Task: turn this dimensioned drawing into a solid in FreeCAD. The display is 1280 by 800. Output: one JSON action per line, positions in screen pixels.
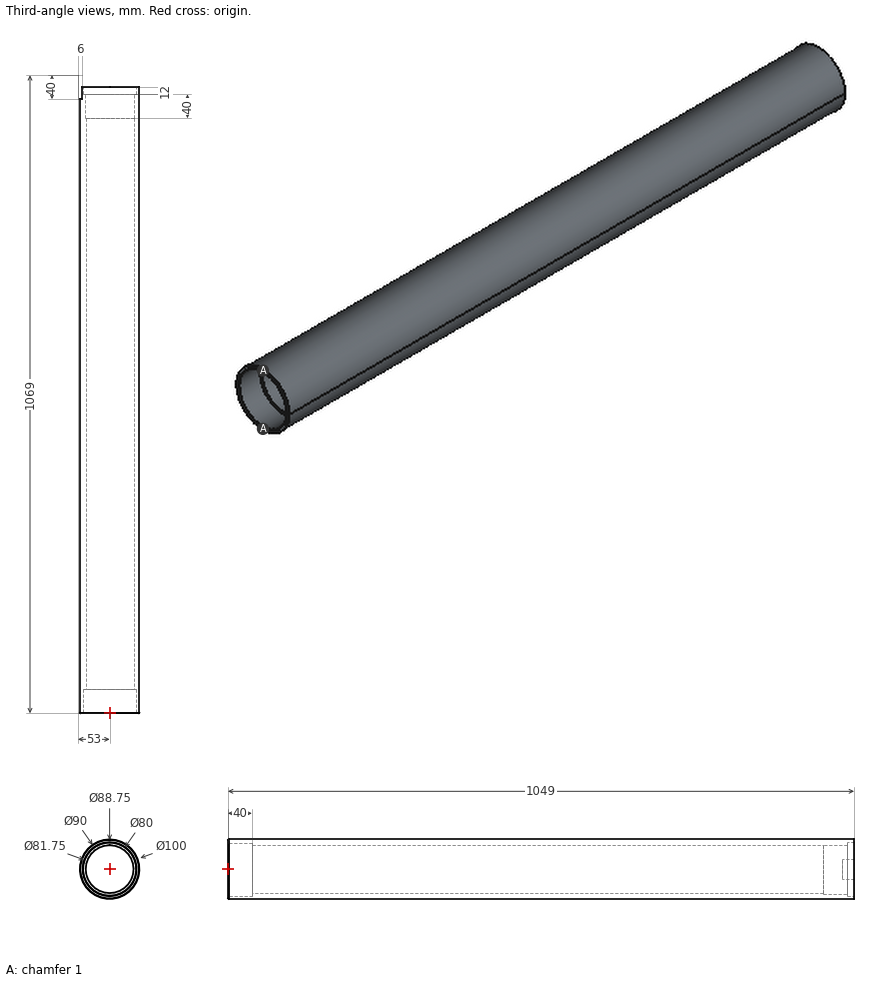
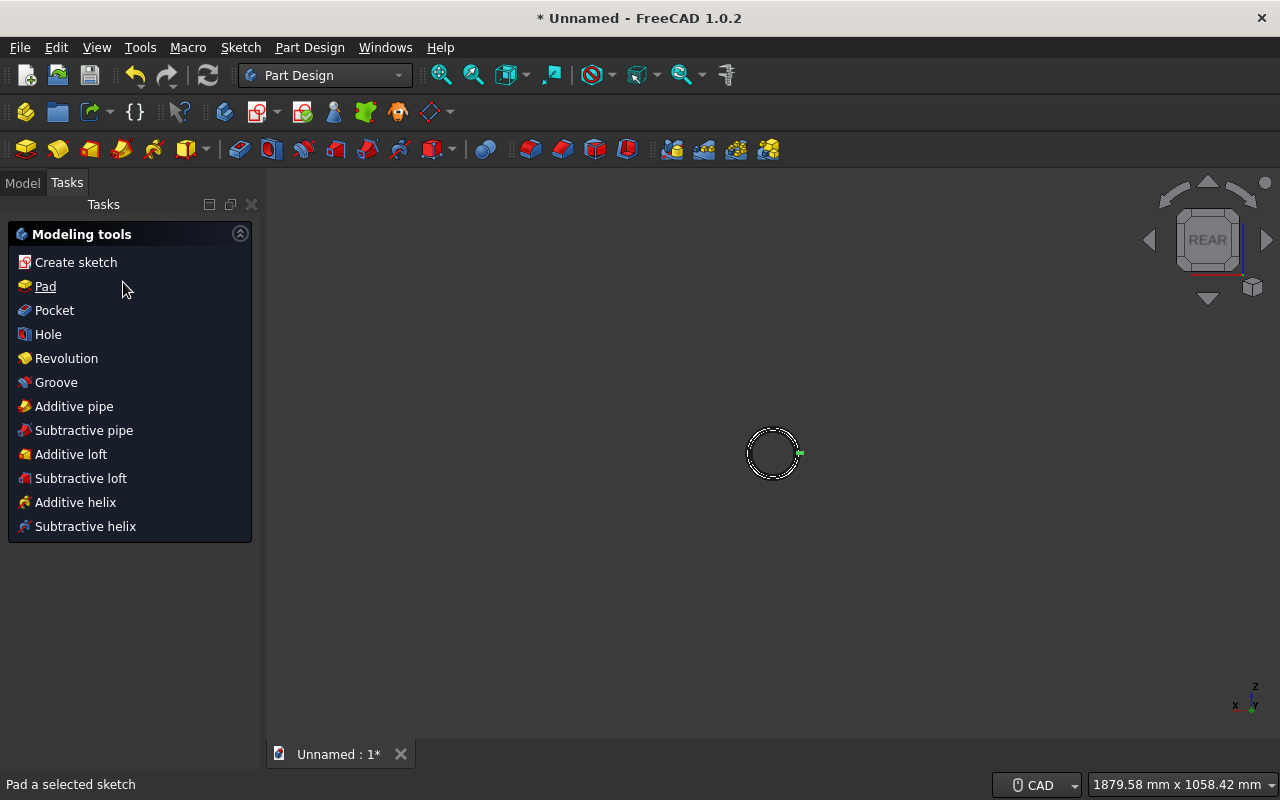
{"action": "left_click", "coordinate": [240, 150]}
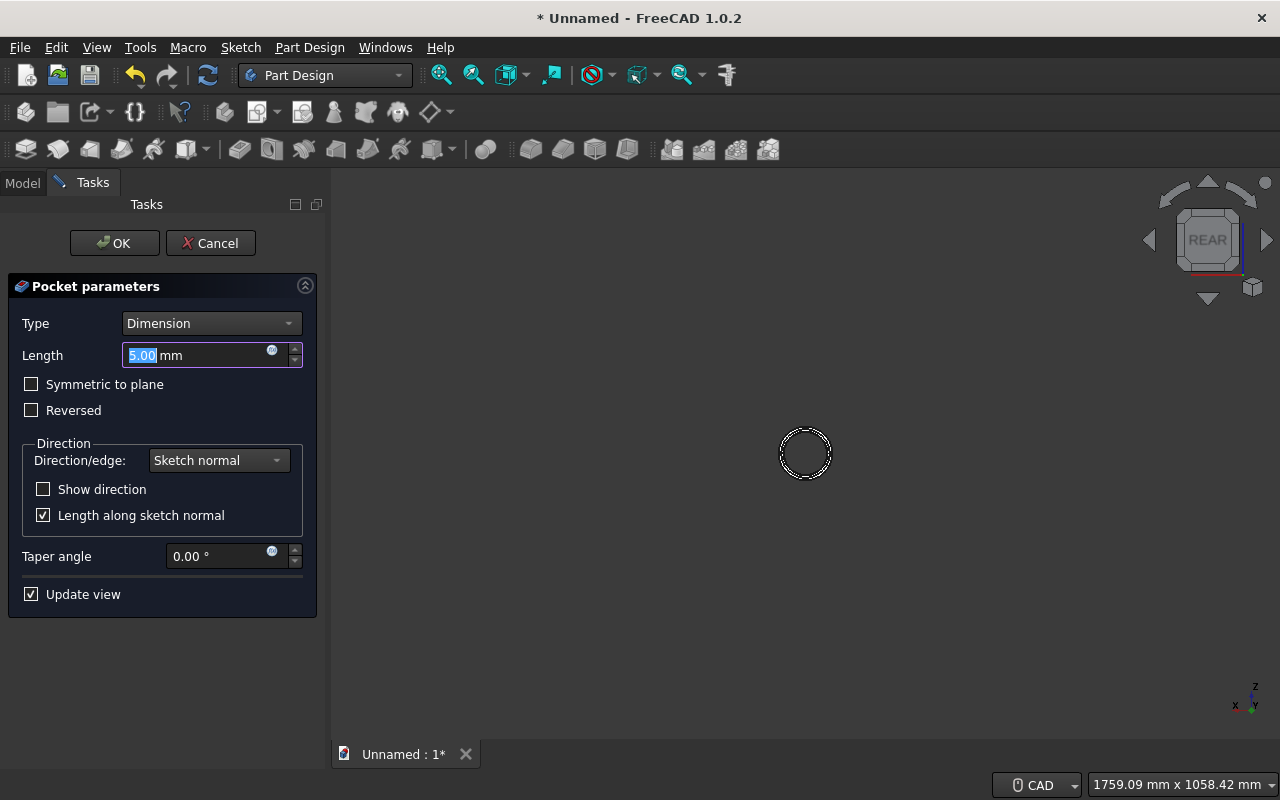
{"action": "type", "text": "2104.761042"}
{"action": "key", "text": "Tab"}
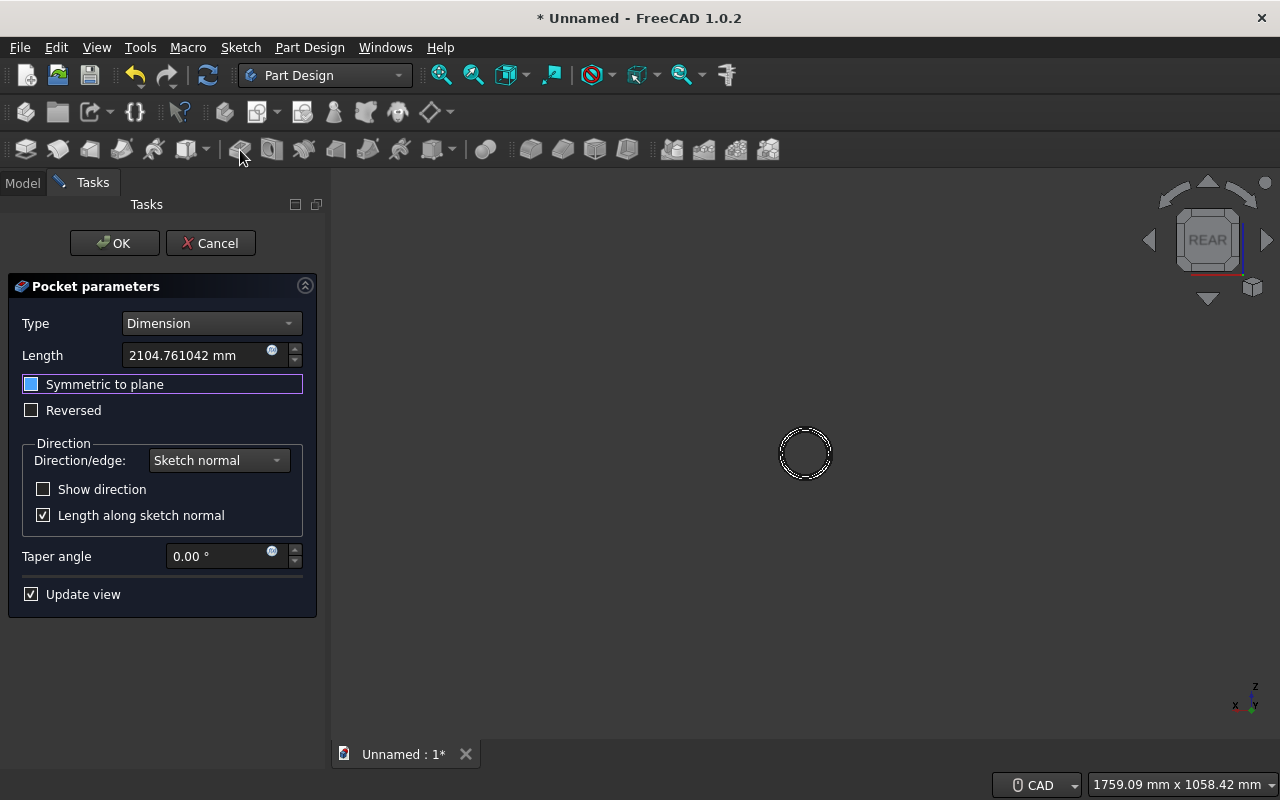
{"action": "left_click", "coordinate": [30, 384]}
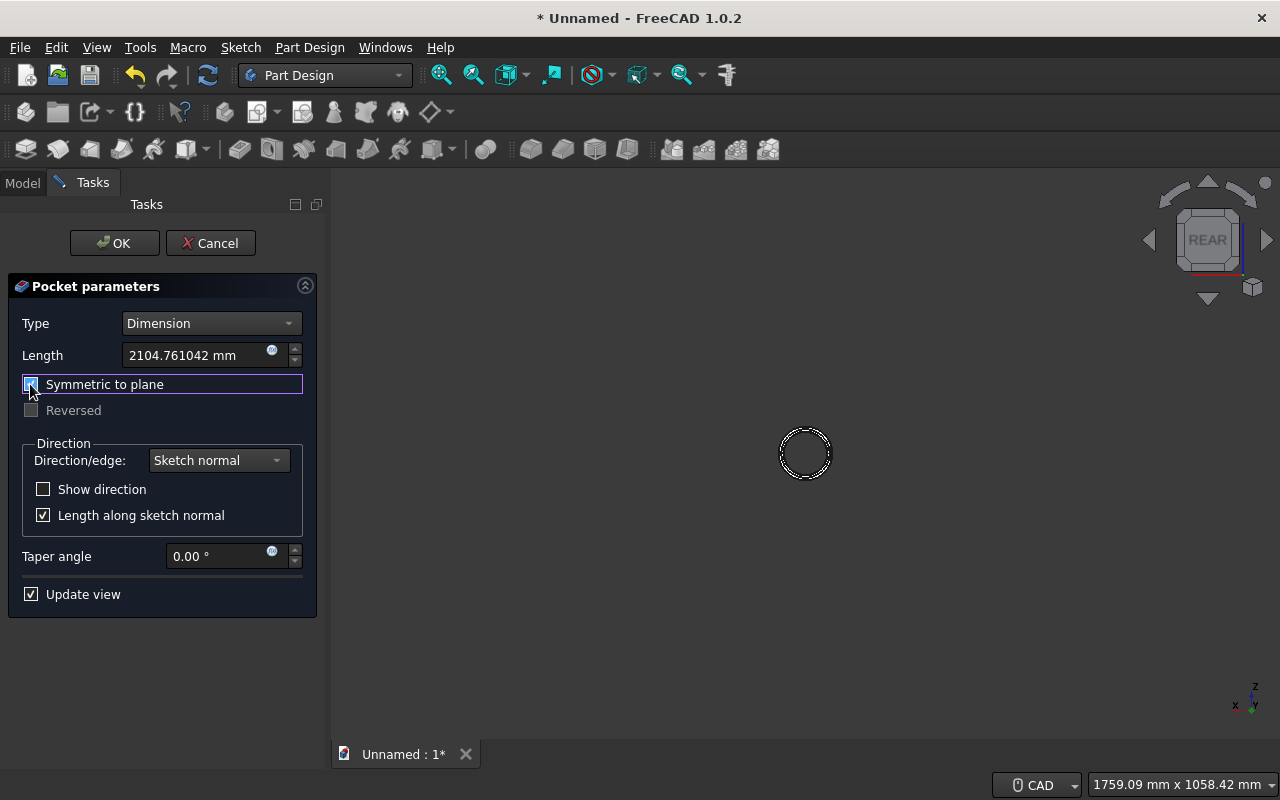
{"action": "left_click", "coordinate": [115, 243]}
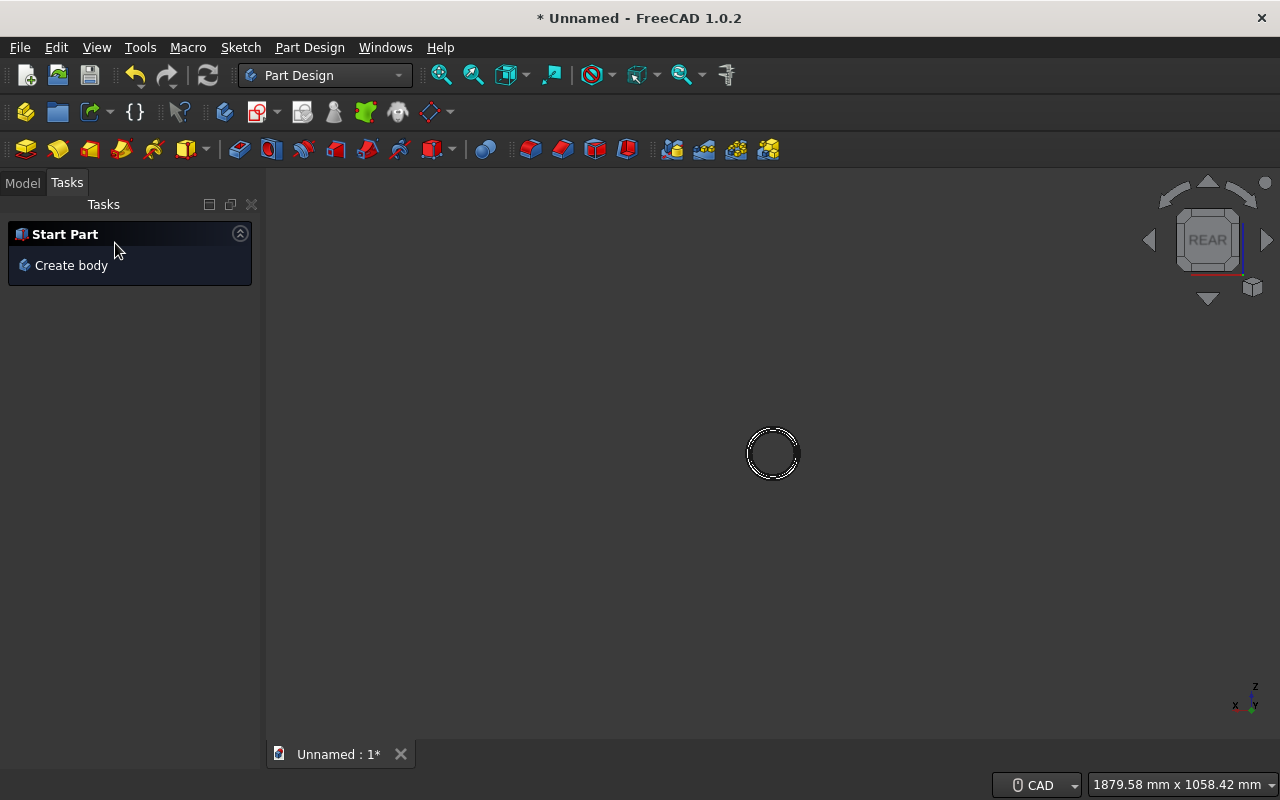
{"action": "key", "text": "0"}